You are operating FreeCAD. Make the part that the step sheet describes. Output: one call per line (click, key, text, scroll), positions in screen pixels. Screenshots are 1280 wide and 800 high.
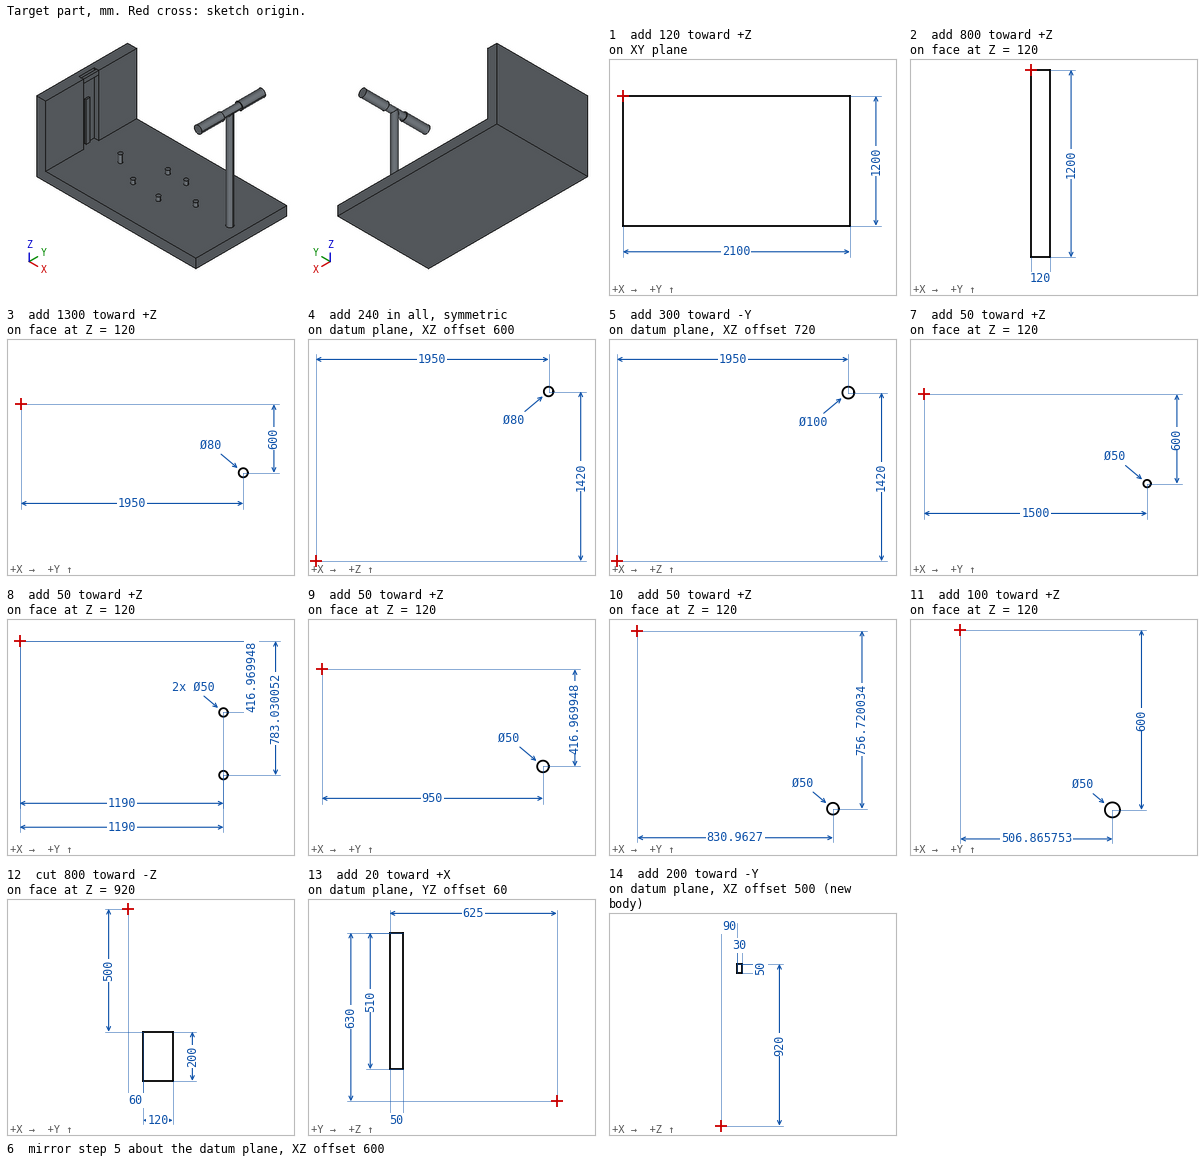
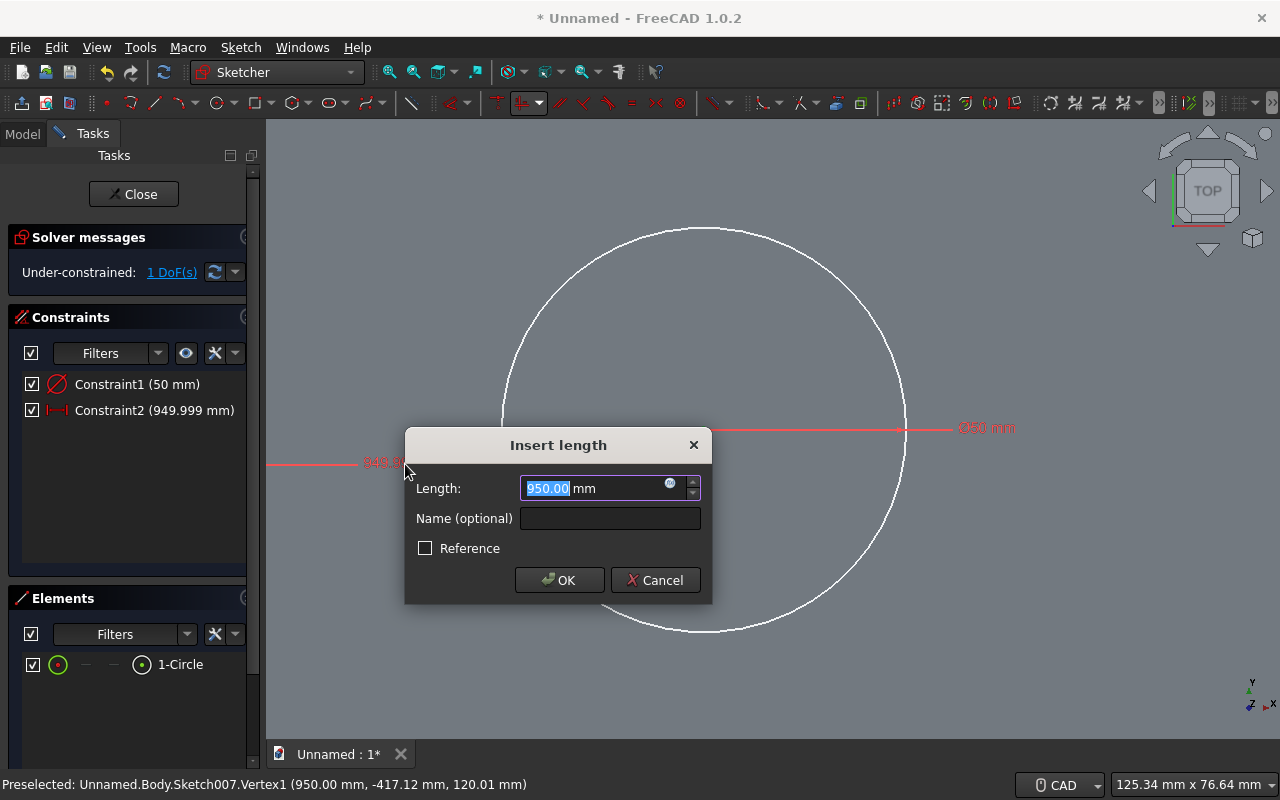
text(950)
key(Return)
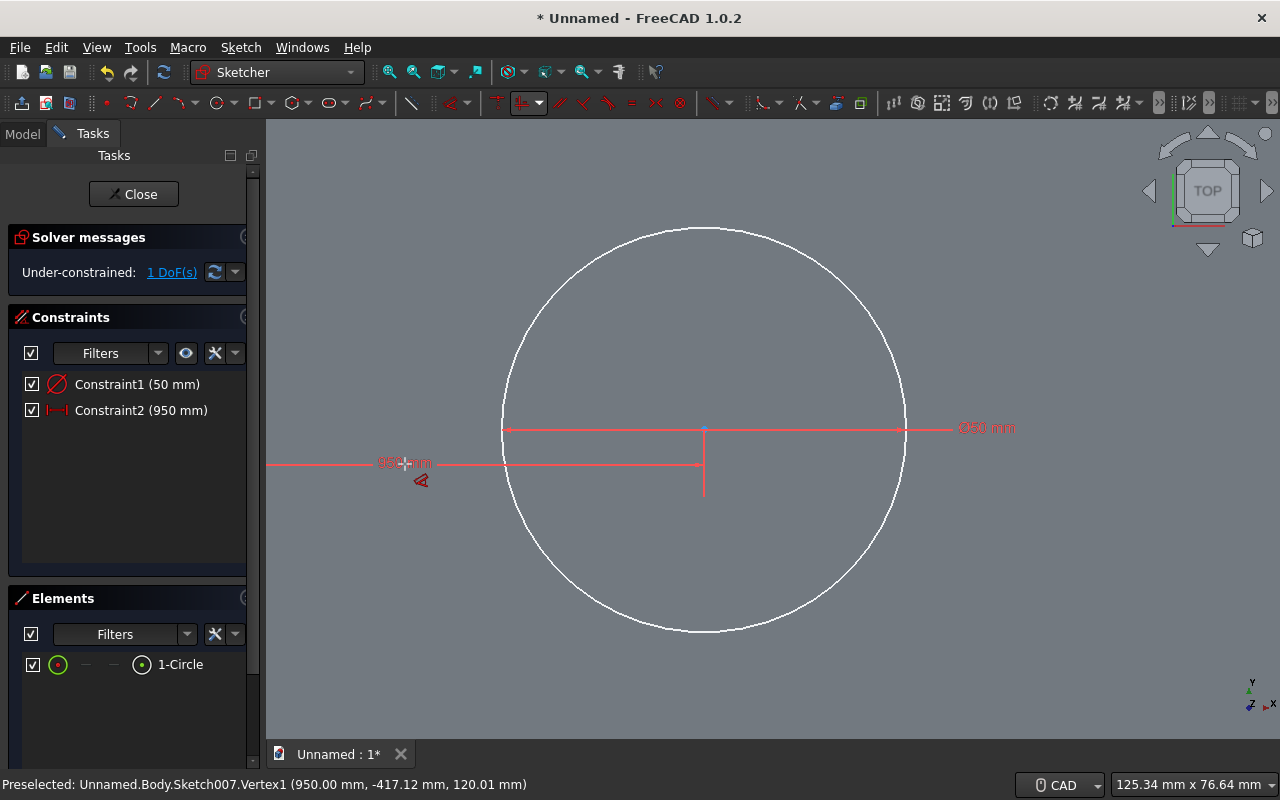
click(704, 430)
click(738, 288)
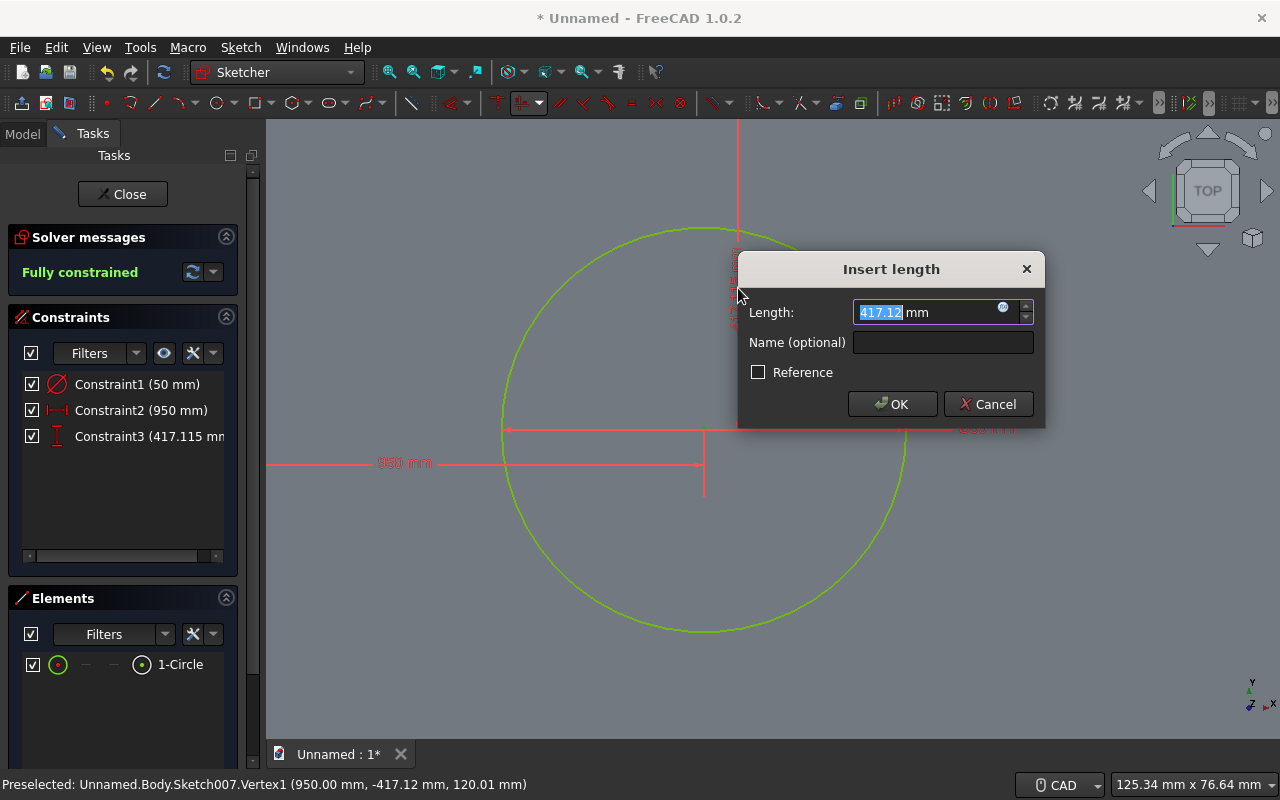
text(416.969948)
key(Return)
key(Escape)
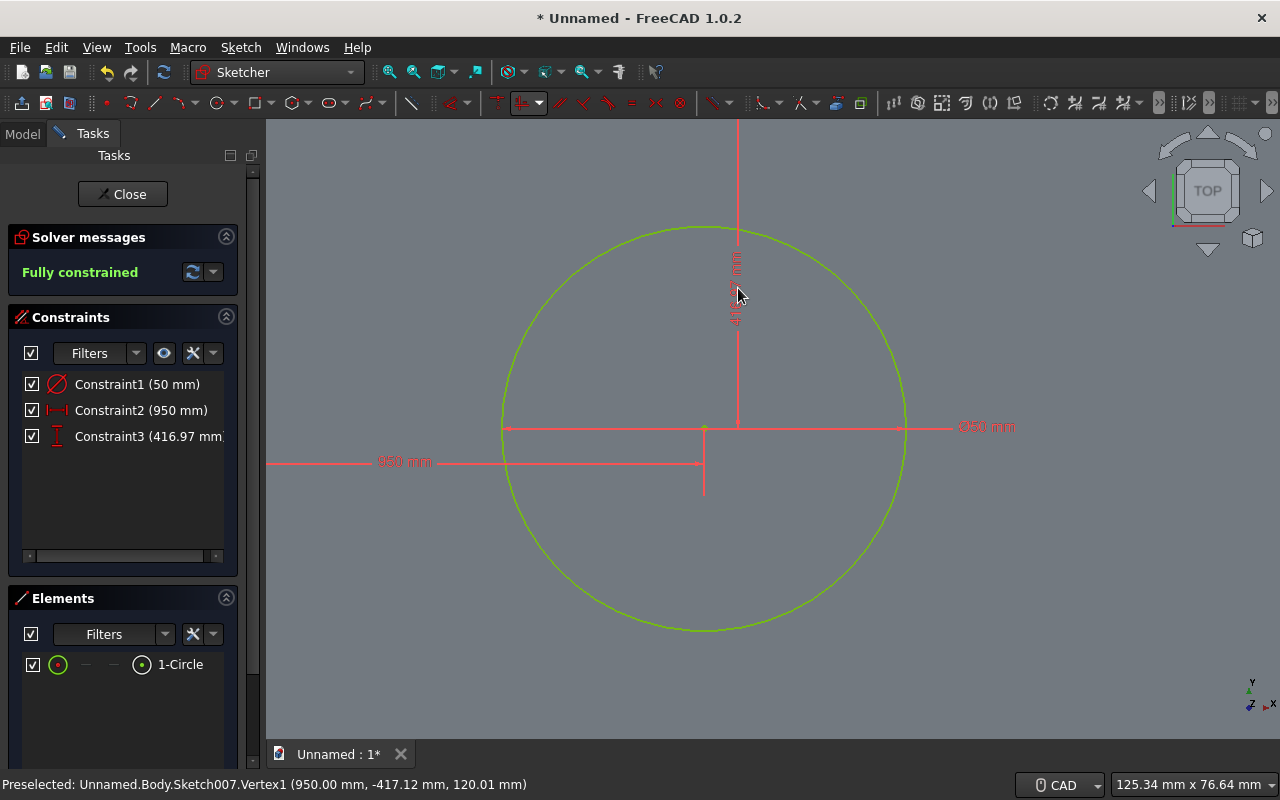
click(123, 194)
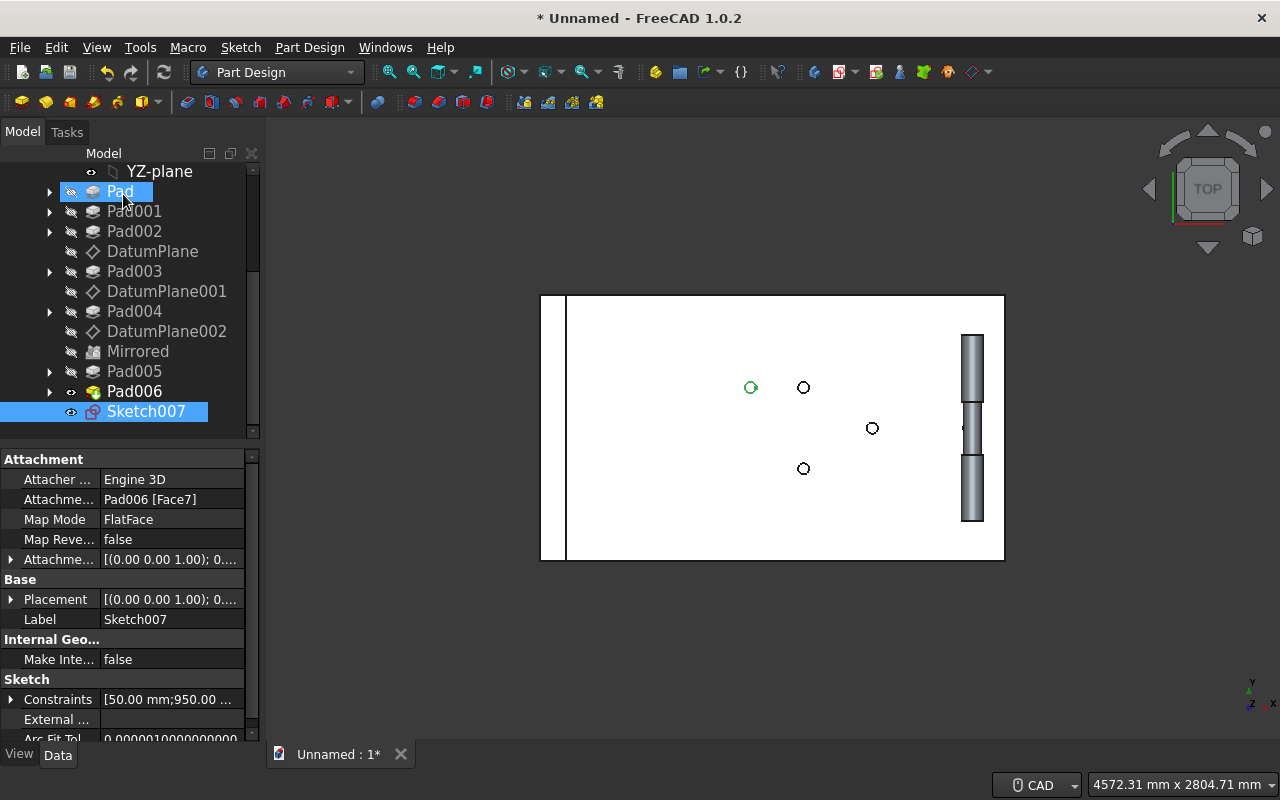
click(22, 102)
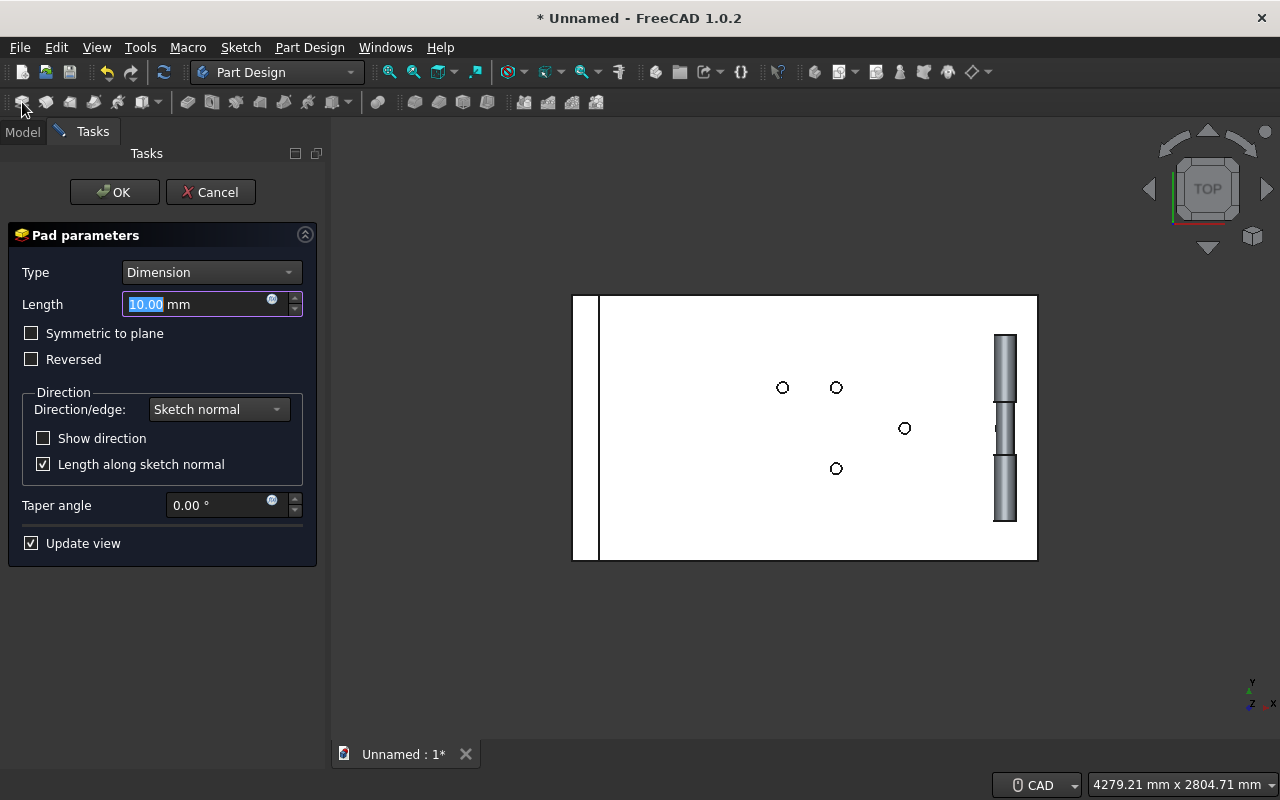
text(50)
key(Tab)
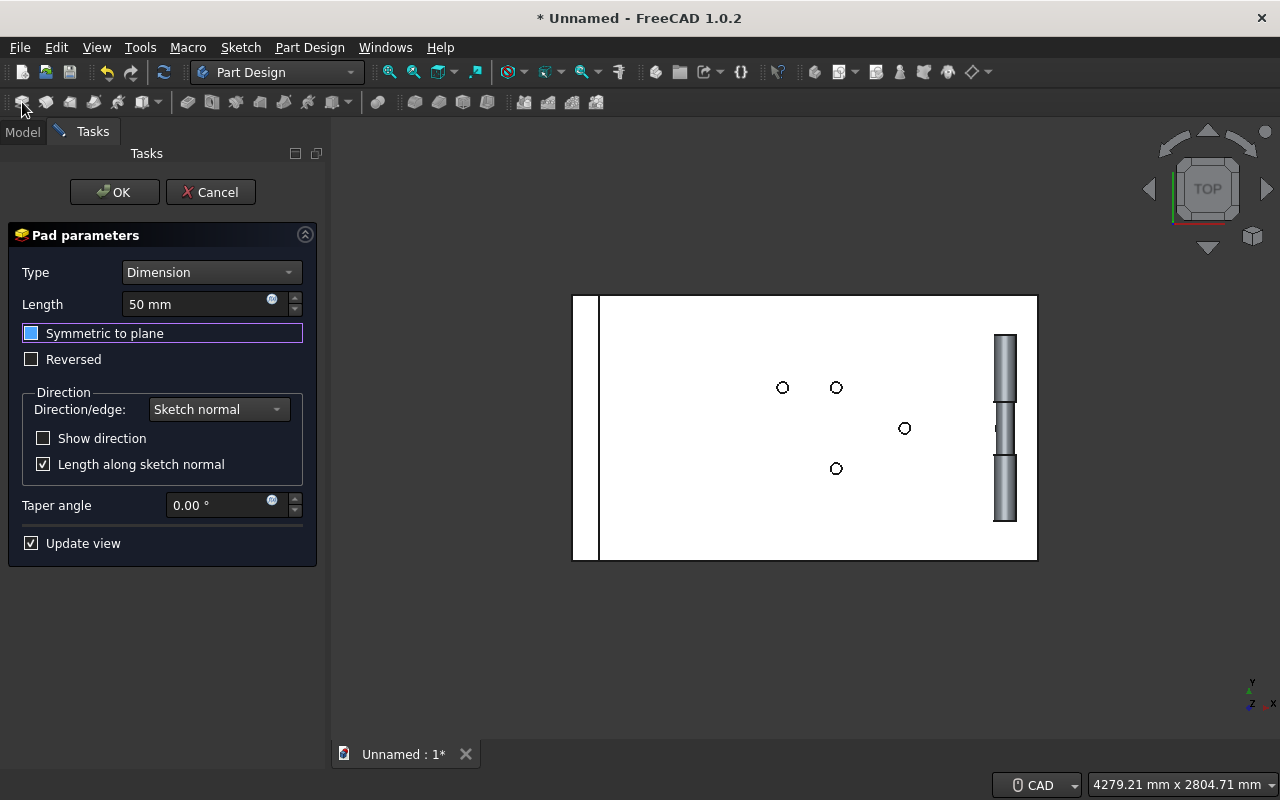
click(115, 192)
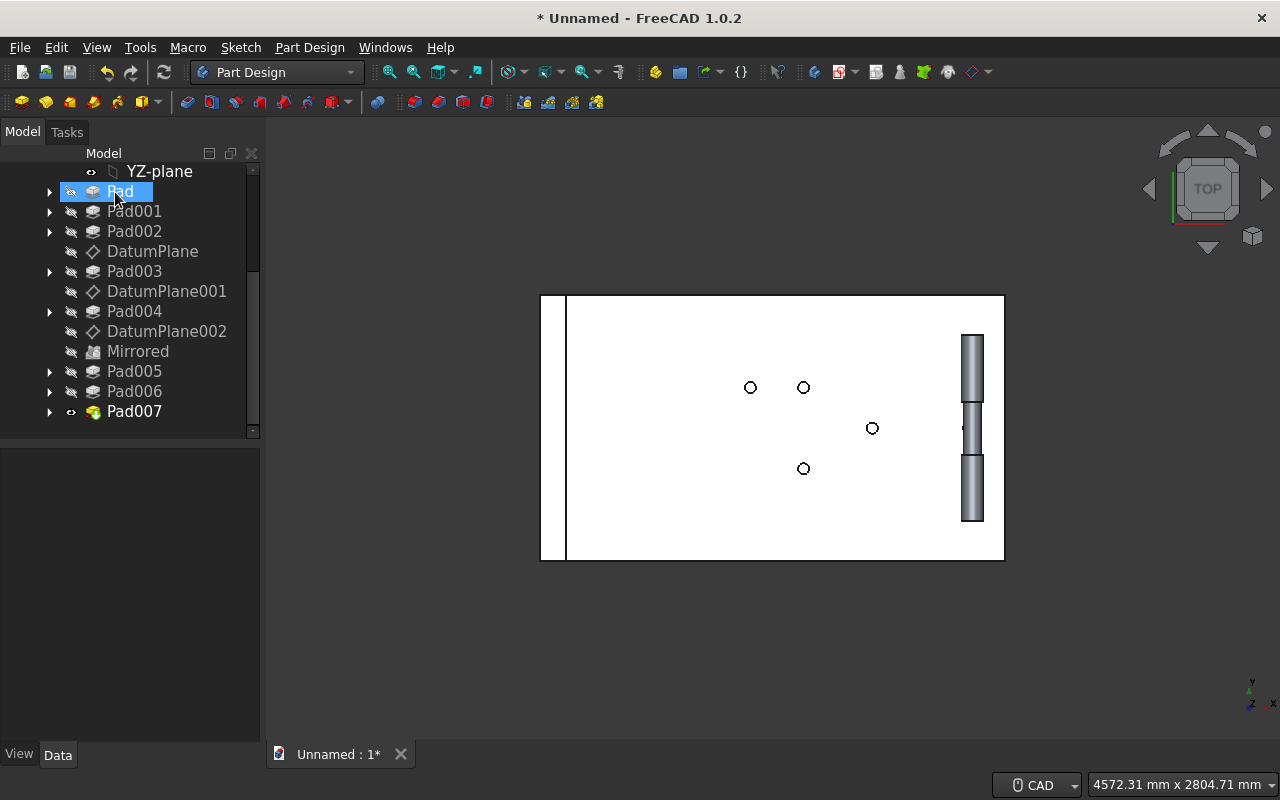
click(660, 465)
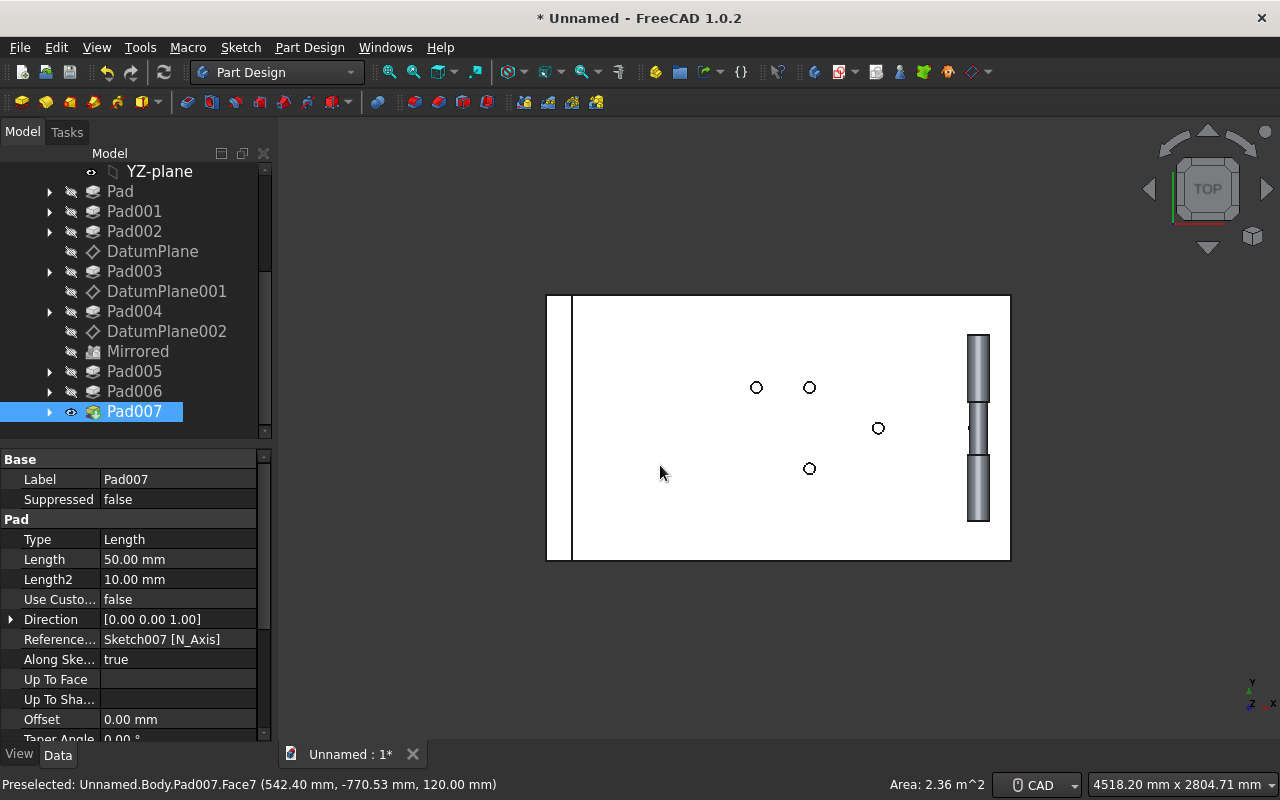
click(840, 72)